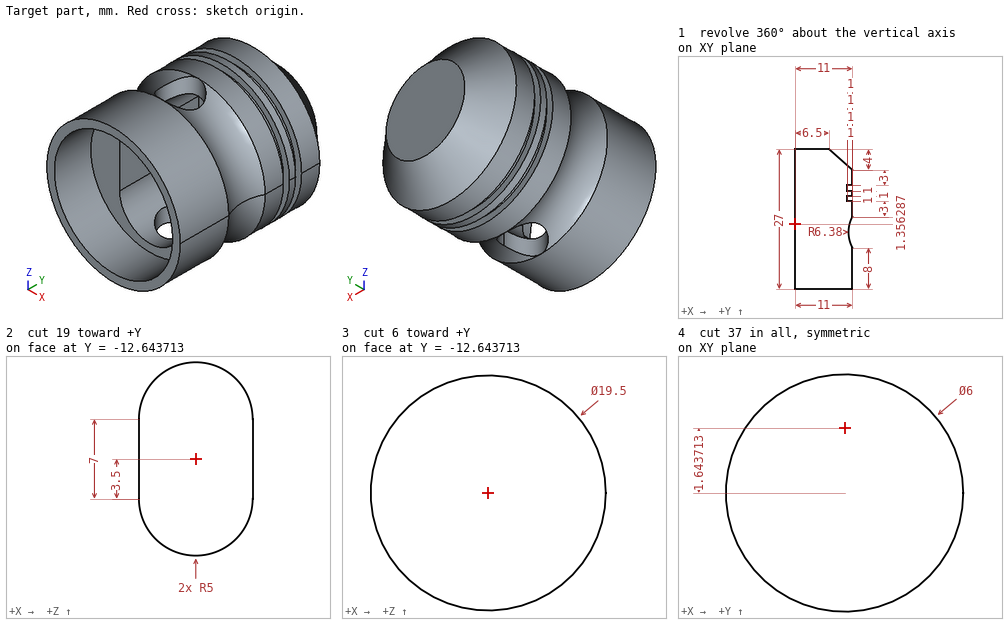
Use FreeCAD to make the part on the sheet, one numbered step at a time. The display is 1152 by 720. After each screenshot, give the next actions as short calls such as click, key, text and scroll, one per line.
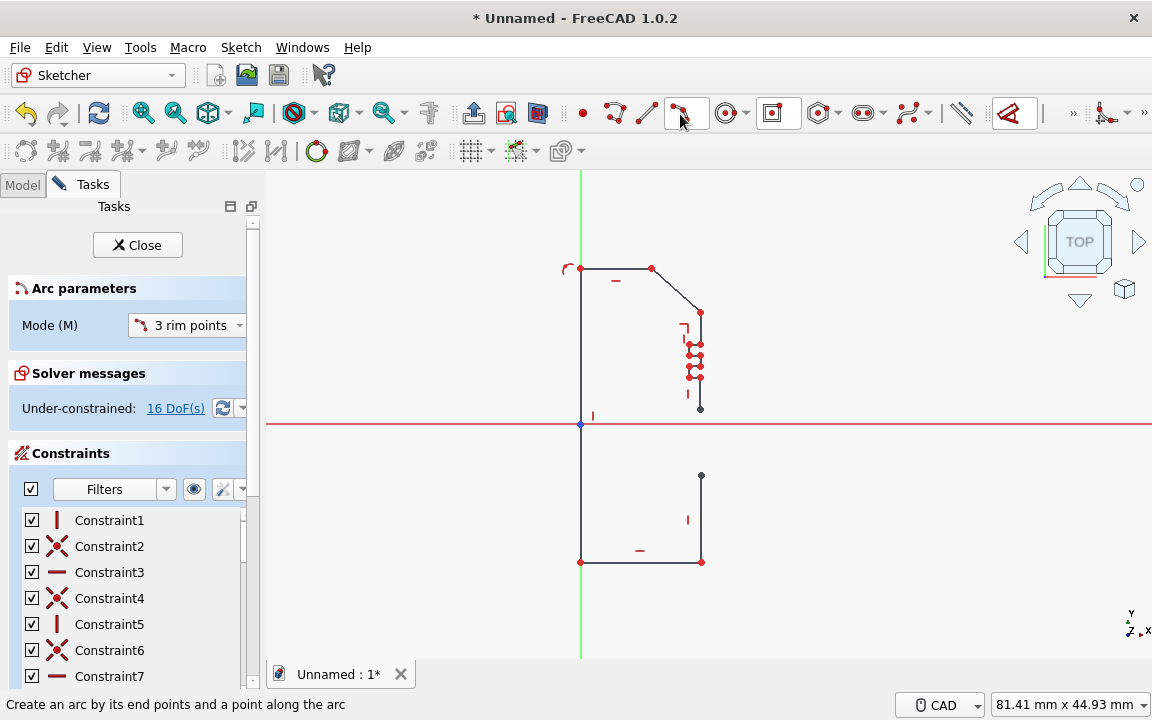
click(701, 476)
click(700, 410)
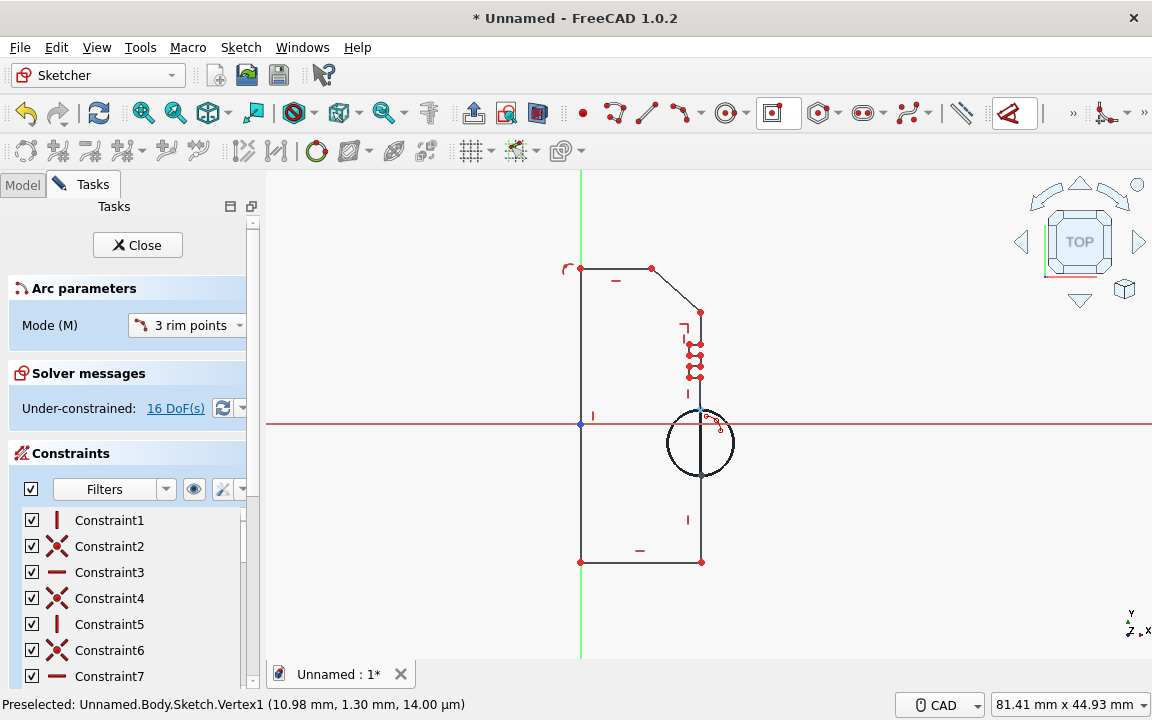
scroll(692, 442, up, 4)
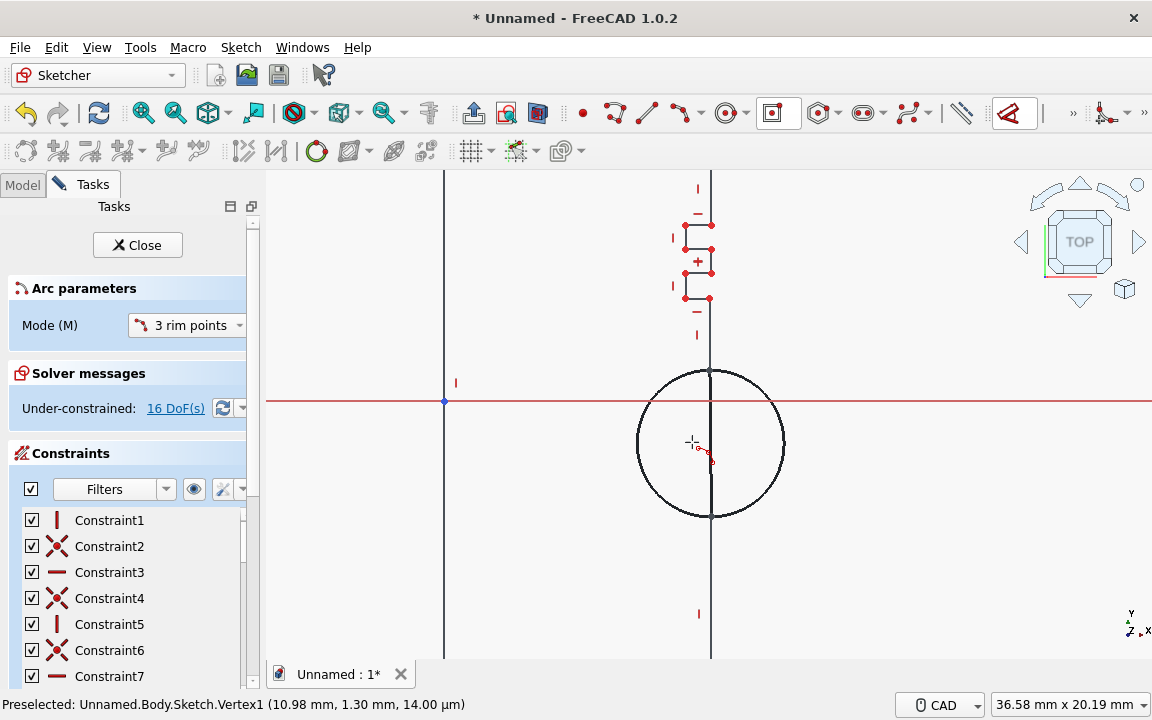
click(692, 441)
key(Escape)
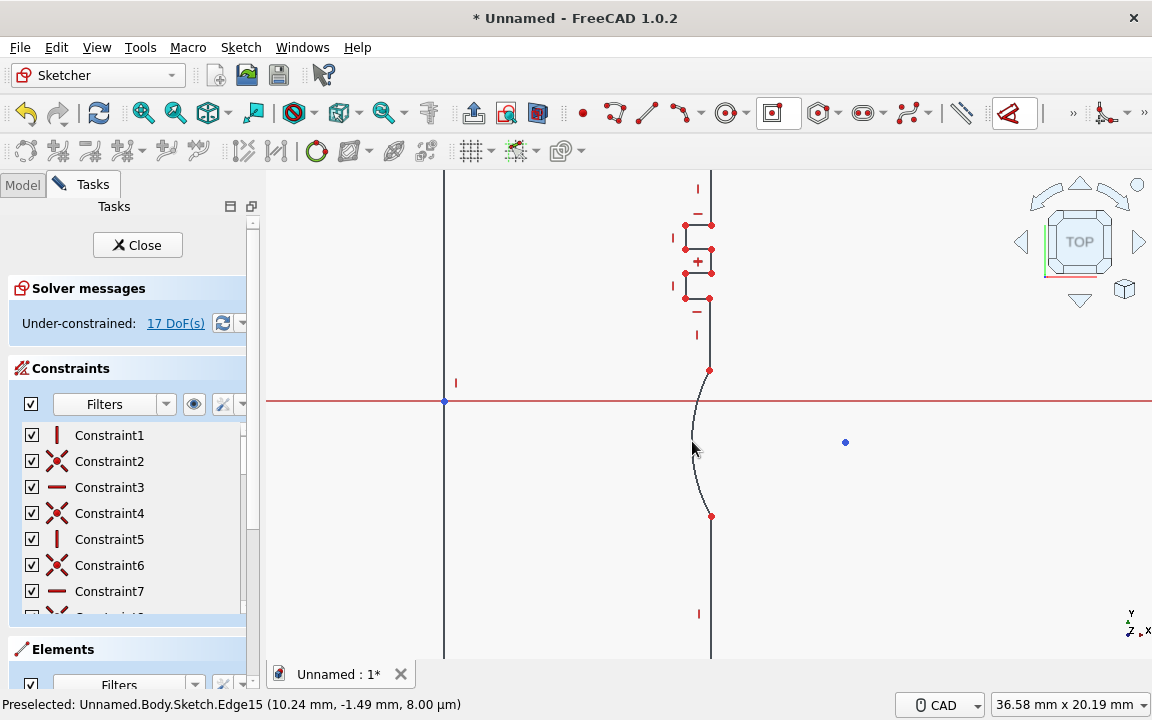
click(695, 413)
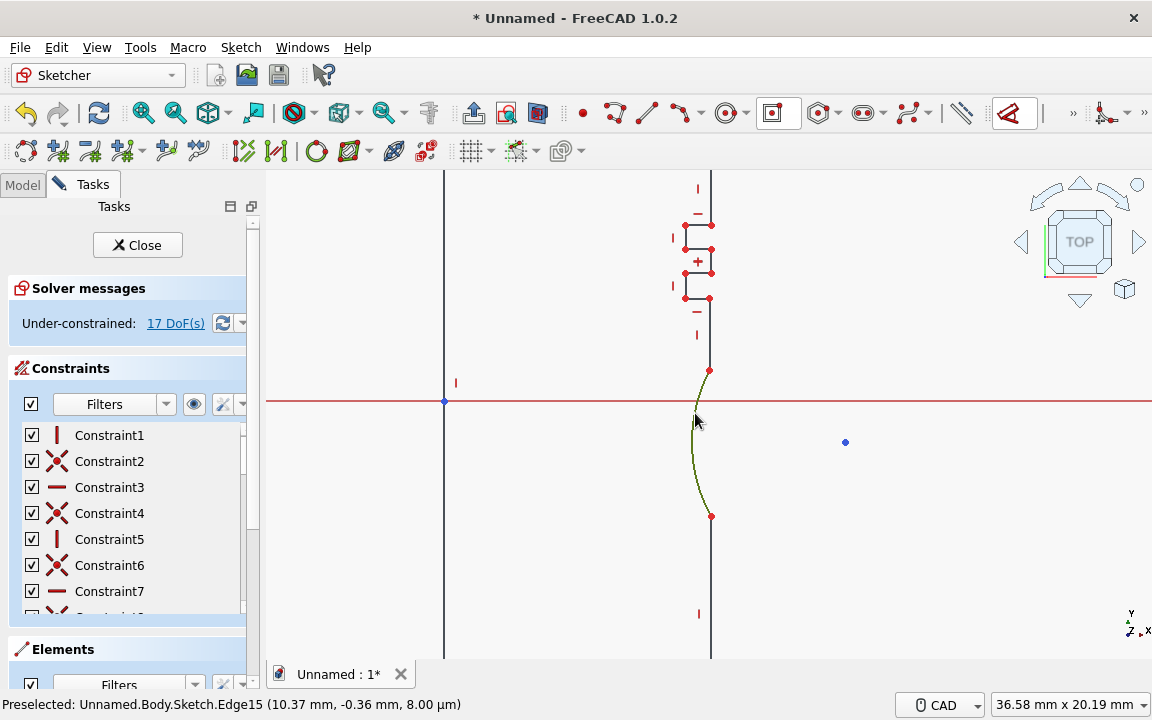
click(1032, 114)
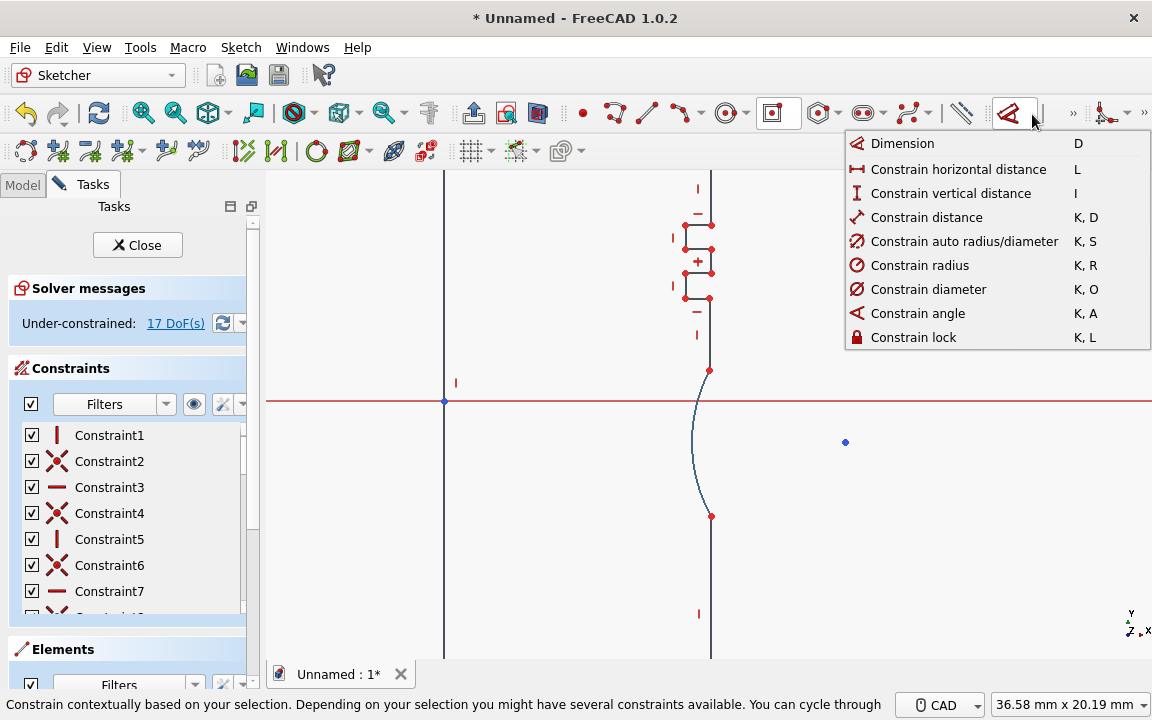
click(998, 265)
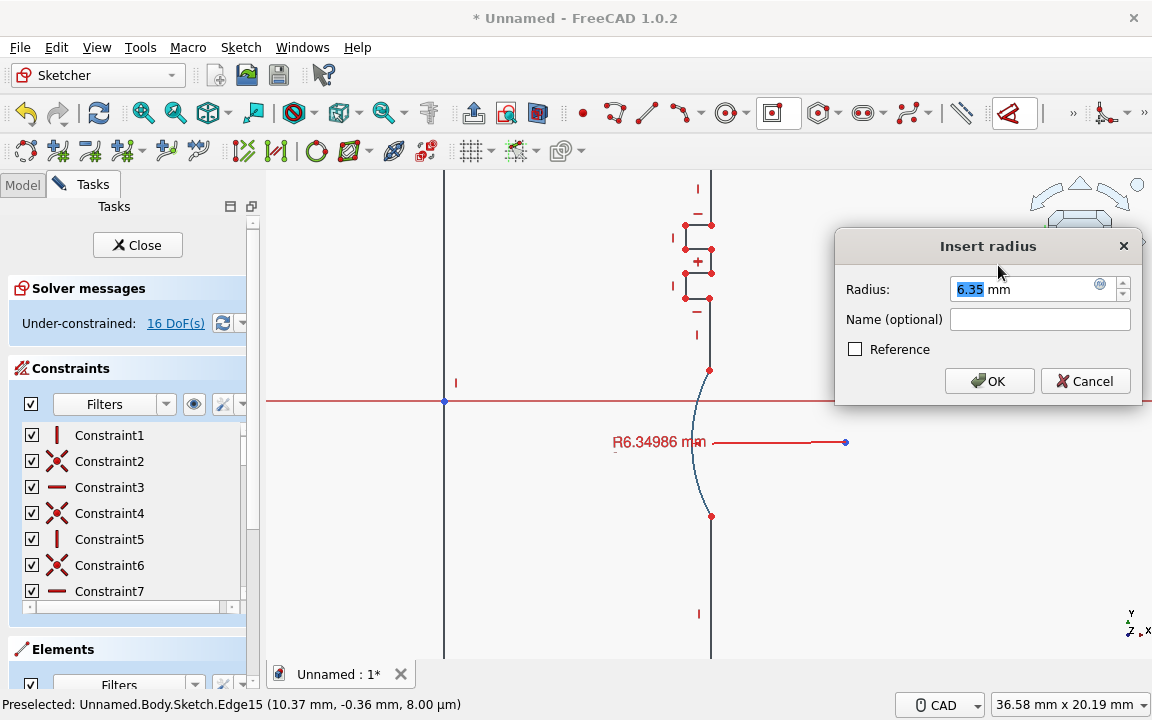
text(6.38)
key(Return)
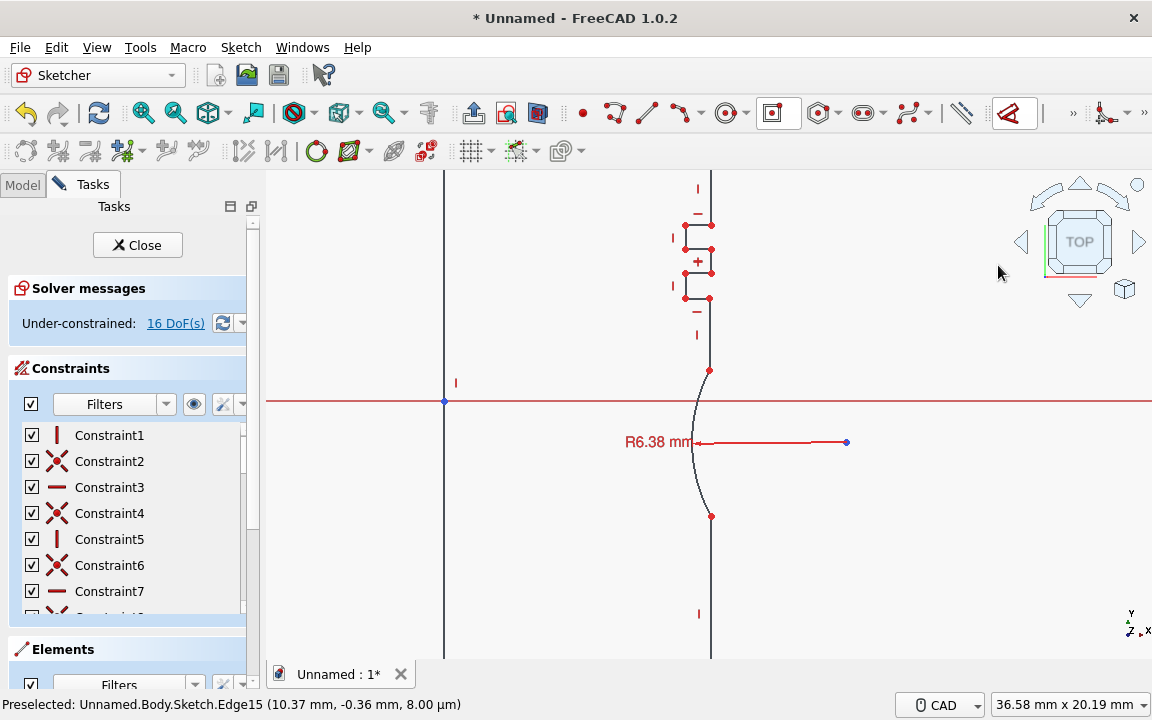
click(710, 349)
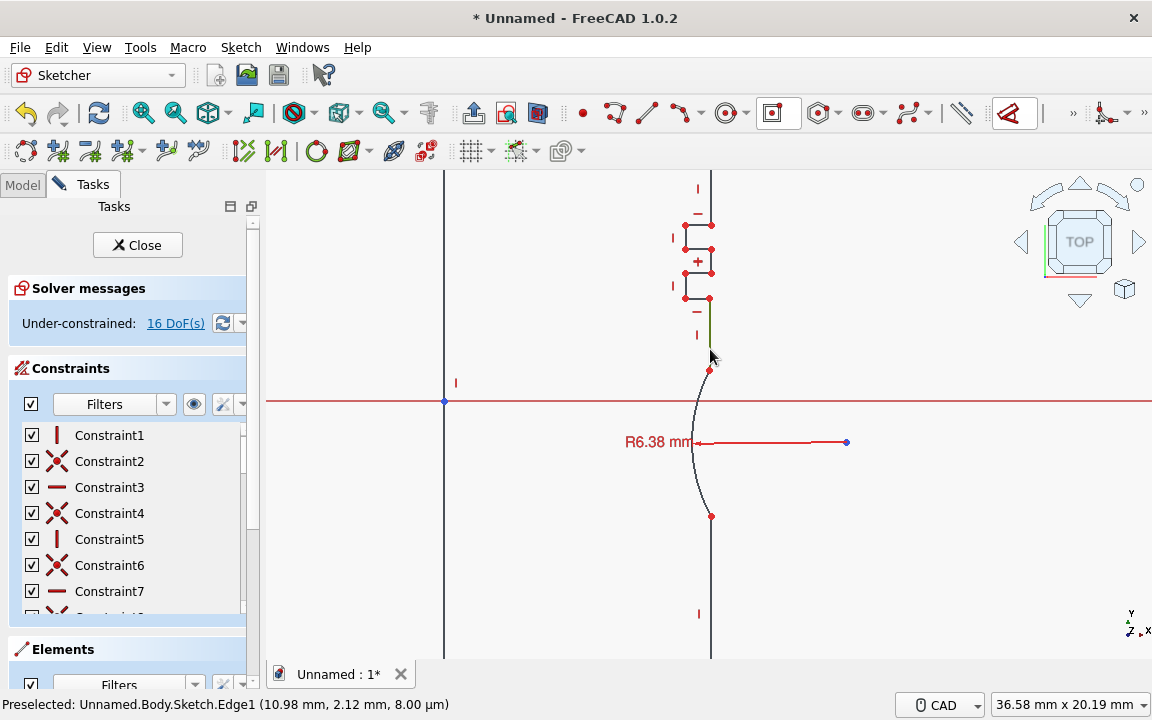
key(i)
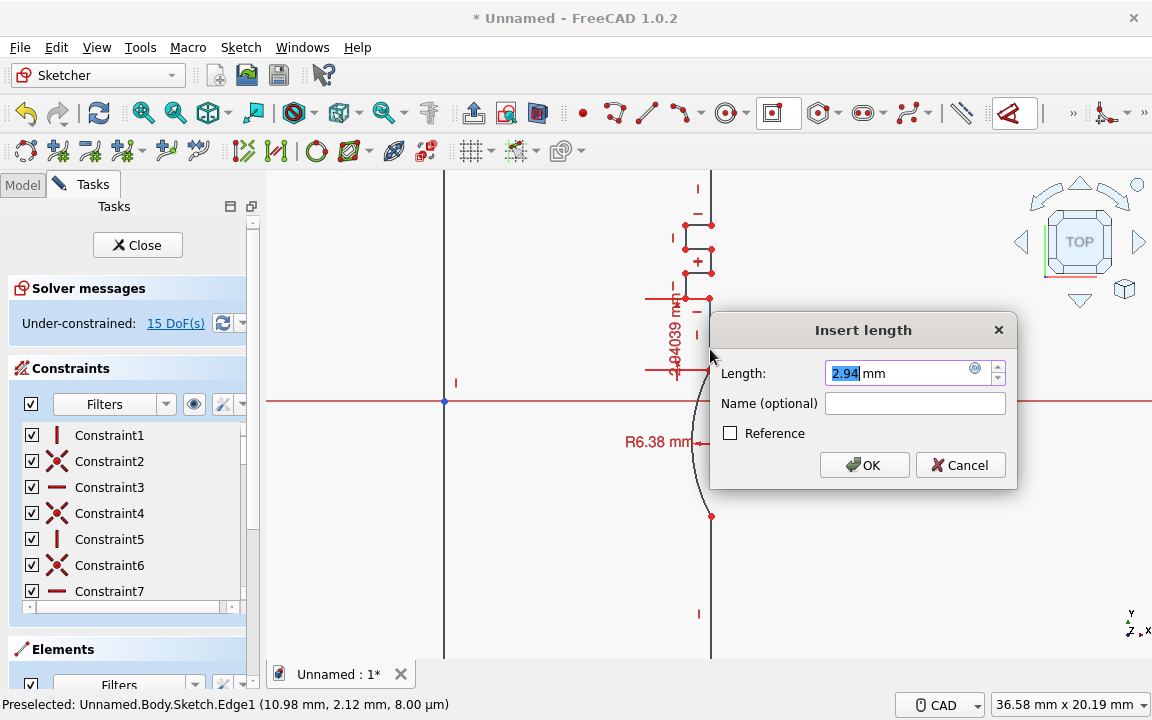
text(3)
key(Return)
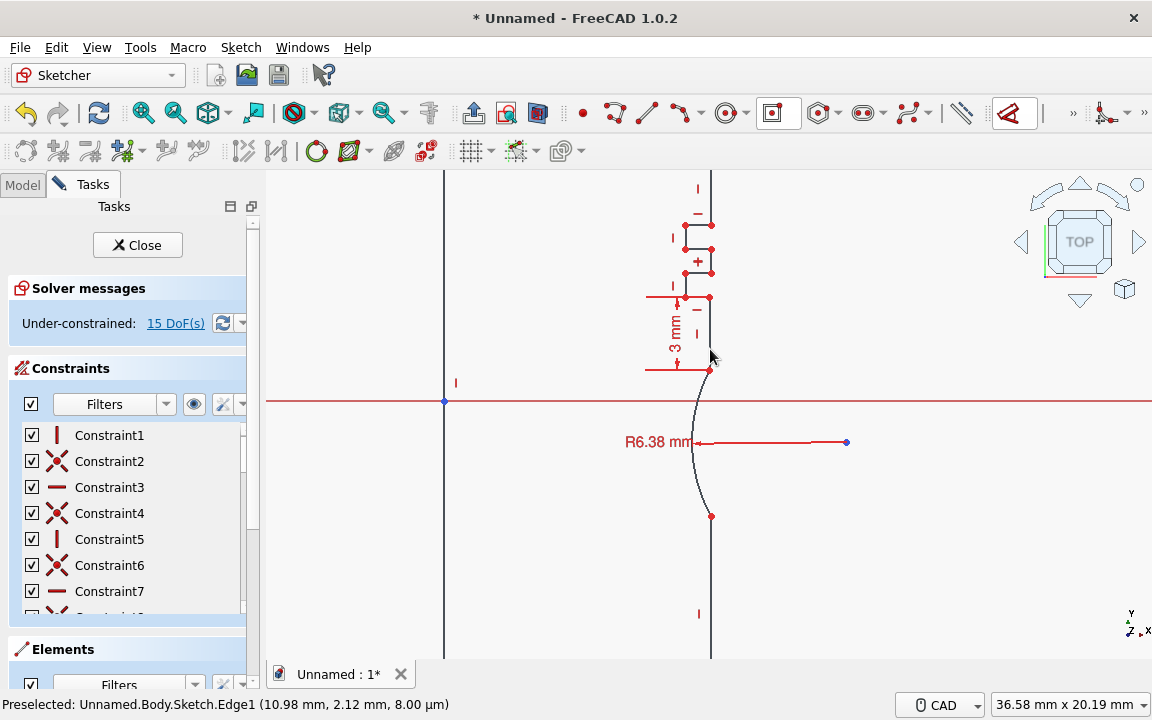
scroll(700, 297, up, 3)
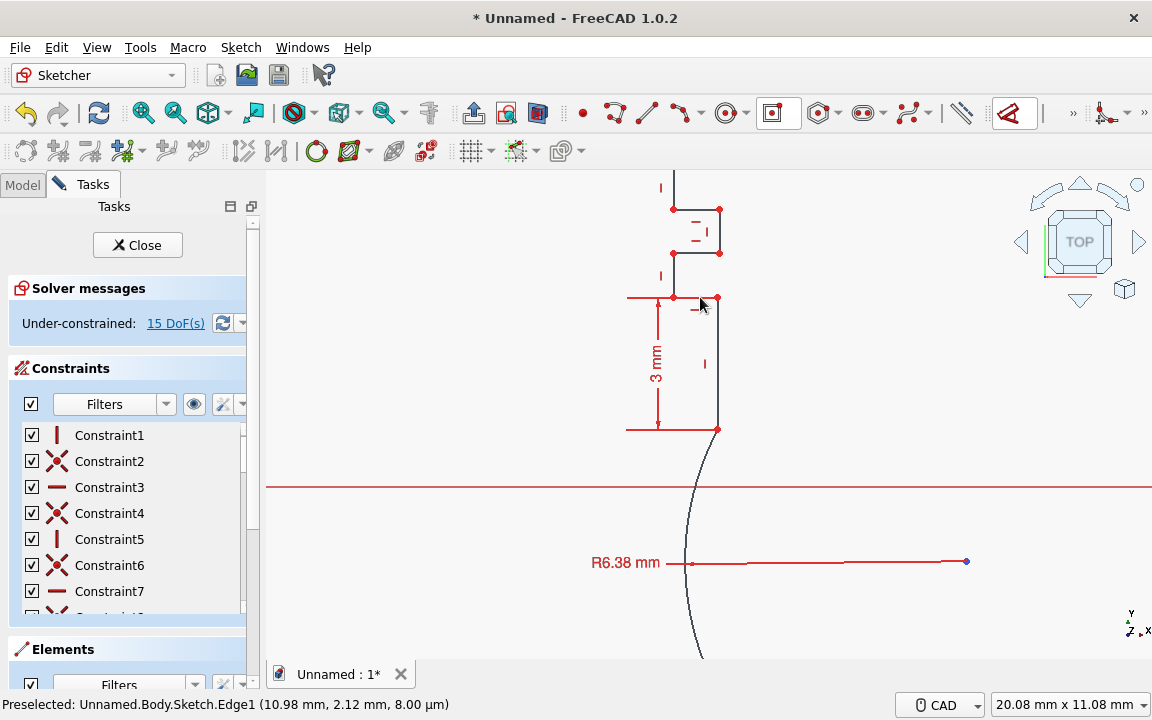
click(700, 298)